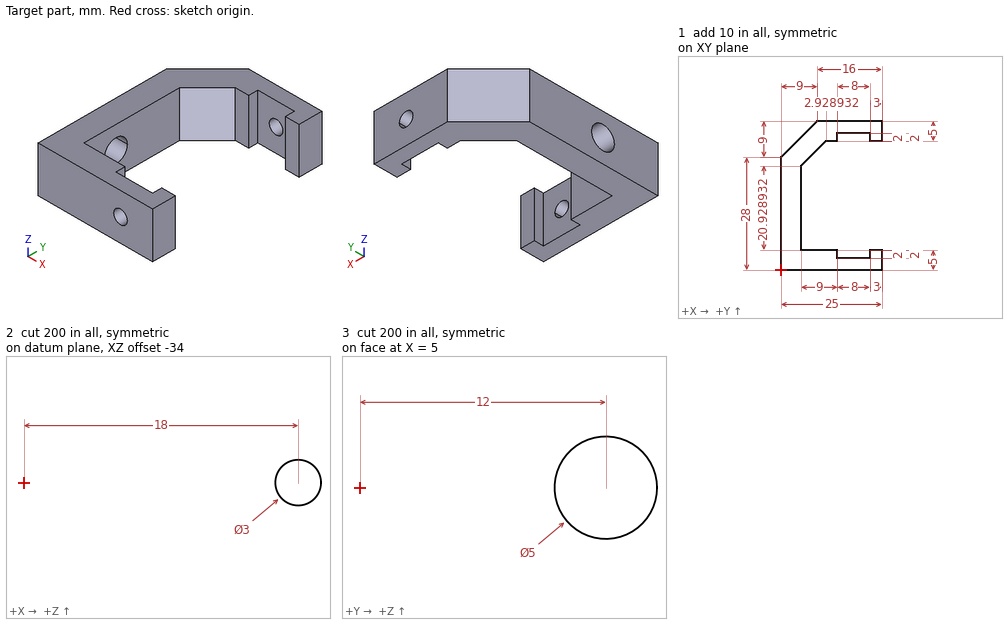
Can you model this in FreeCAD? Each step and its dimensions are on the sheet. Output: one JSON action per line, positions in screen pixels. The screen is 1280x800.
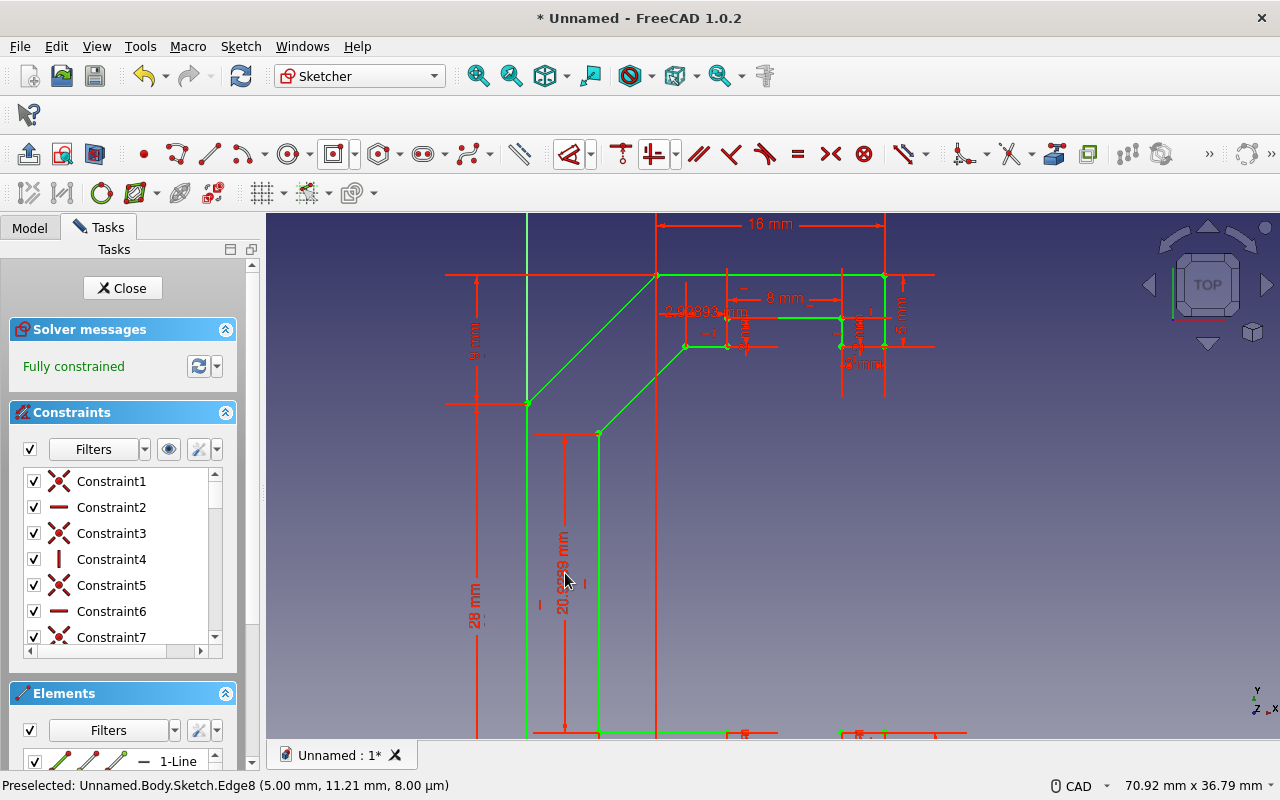
{"action": "left_click", "coordinate": [123, 288]}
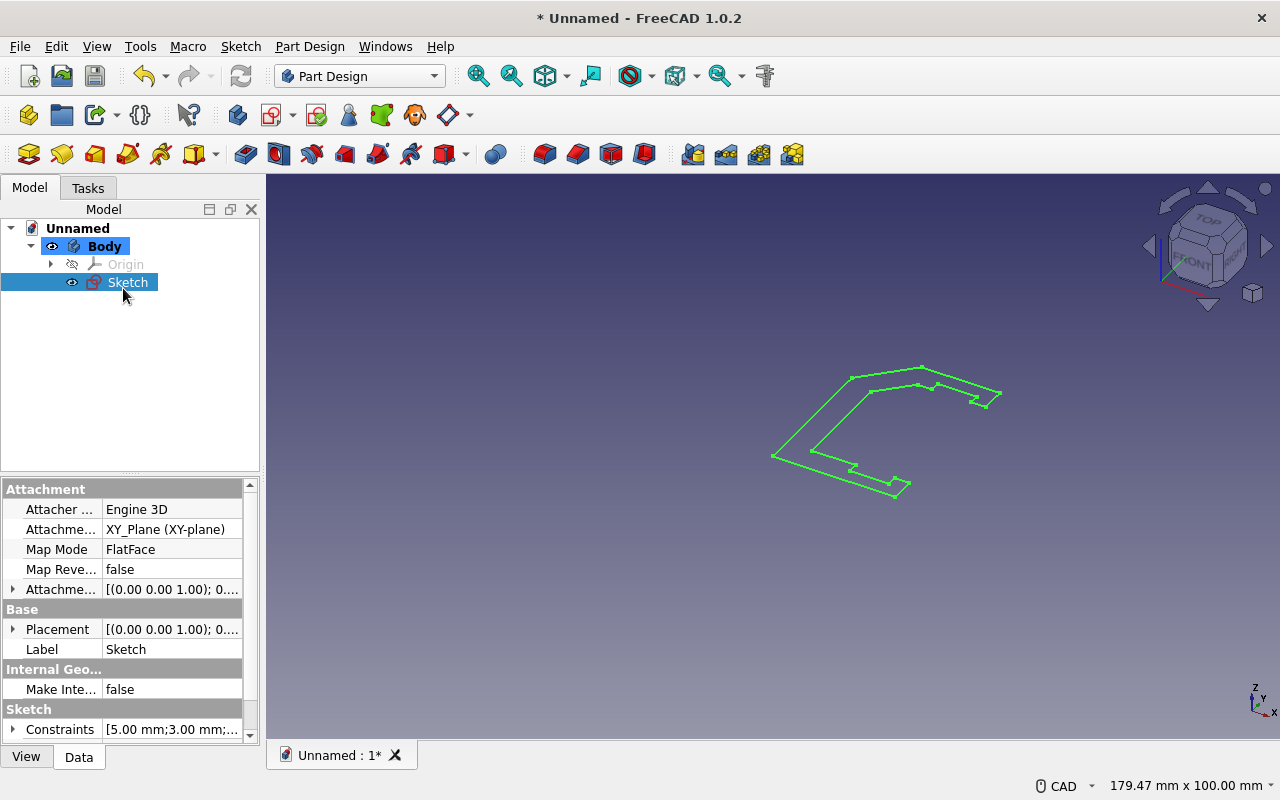
{"action": "left_click", "coordinate": [29, 154]}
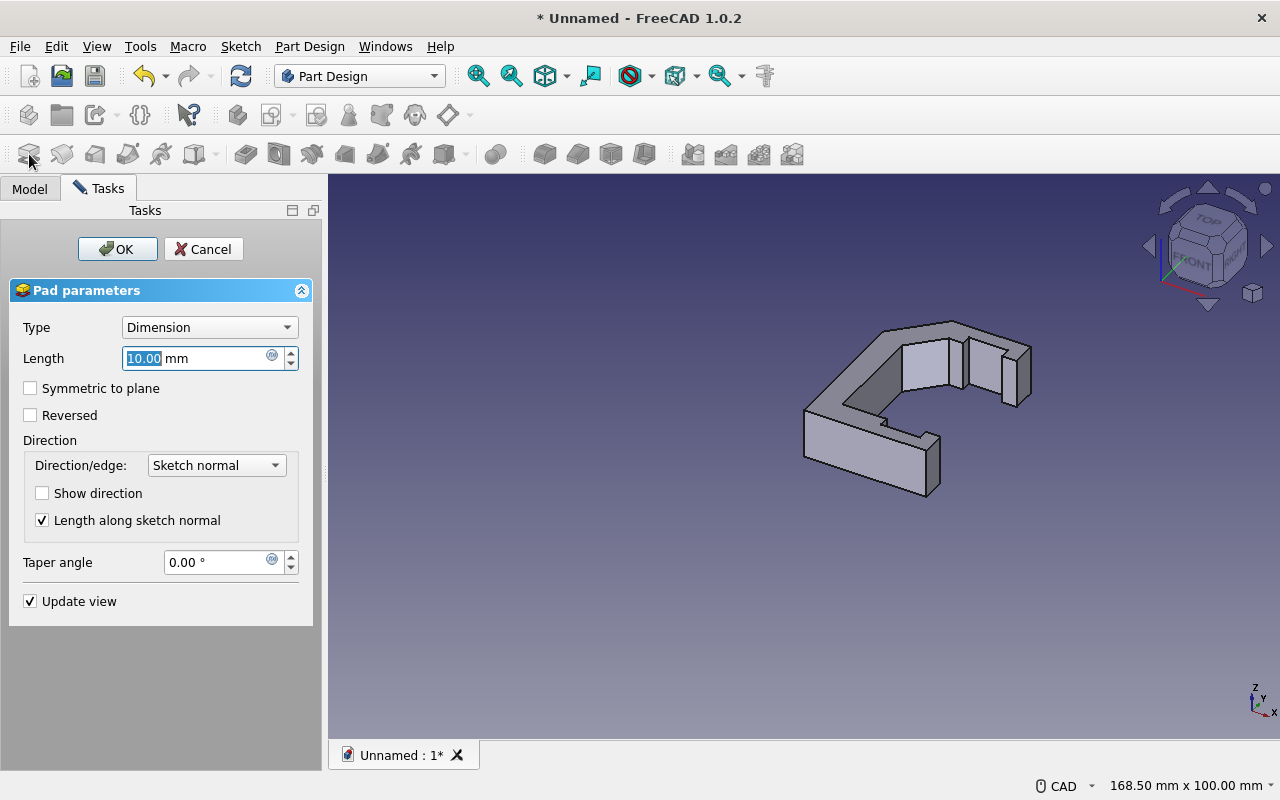
{"action": "type", "text": "10"}
{"action": "key", "text": "Tab"}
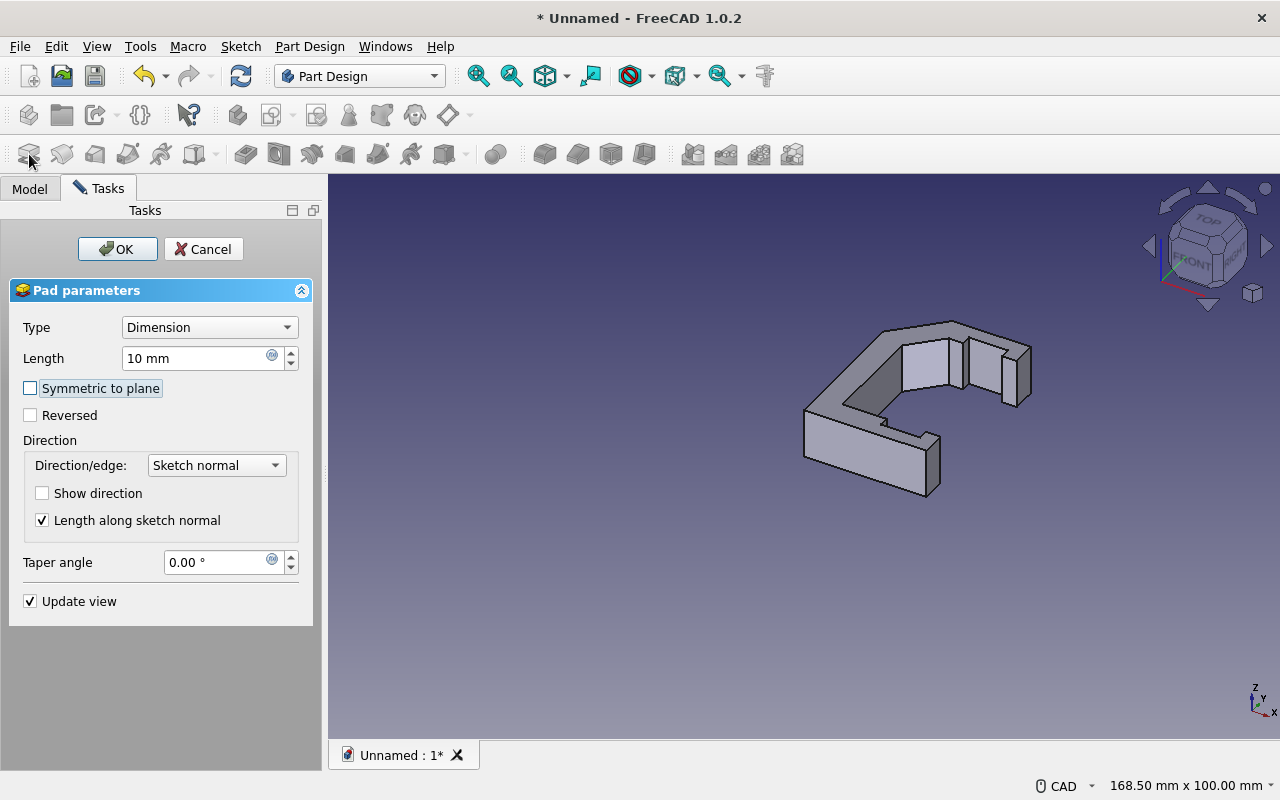
{"action": "left_click", "coordinate": [31, 388]}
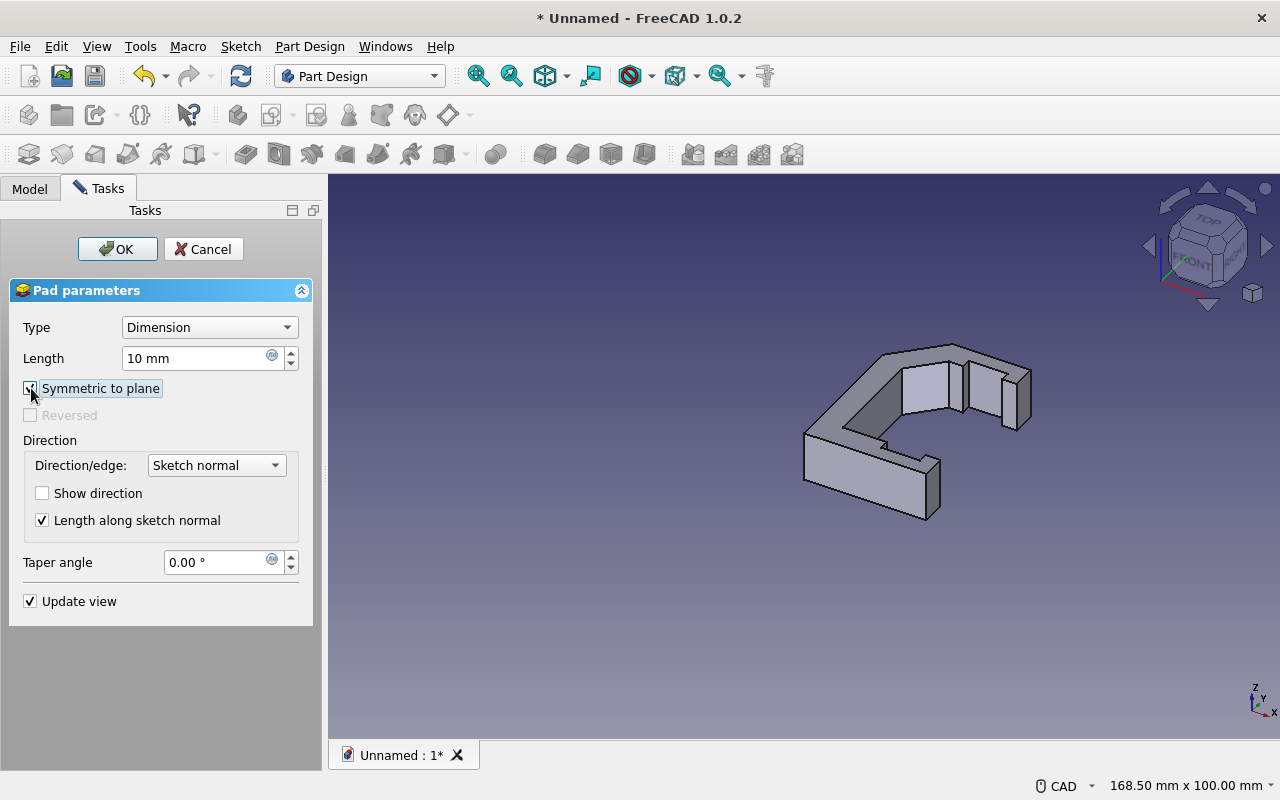
{"action": "left_click", "coordinate": [118, 249]}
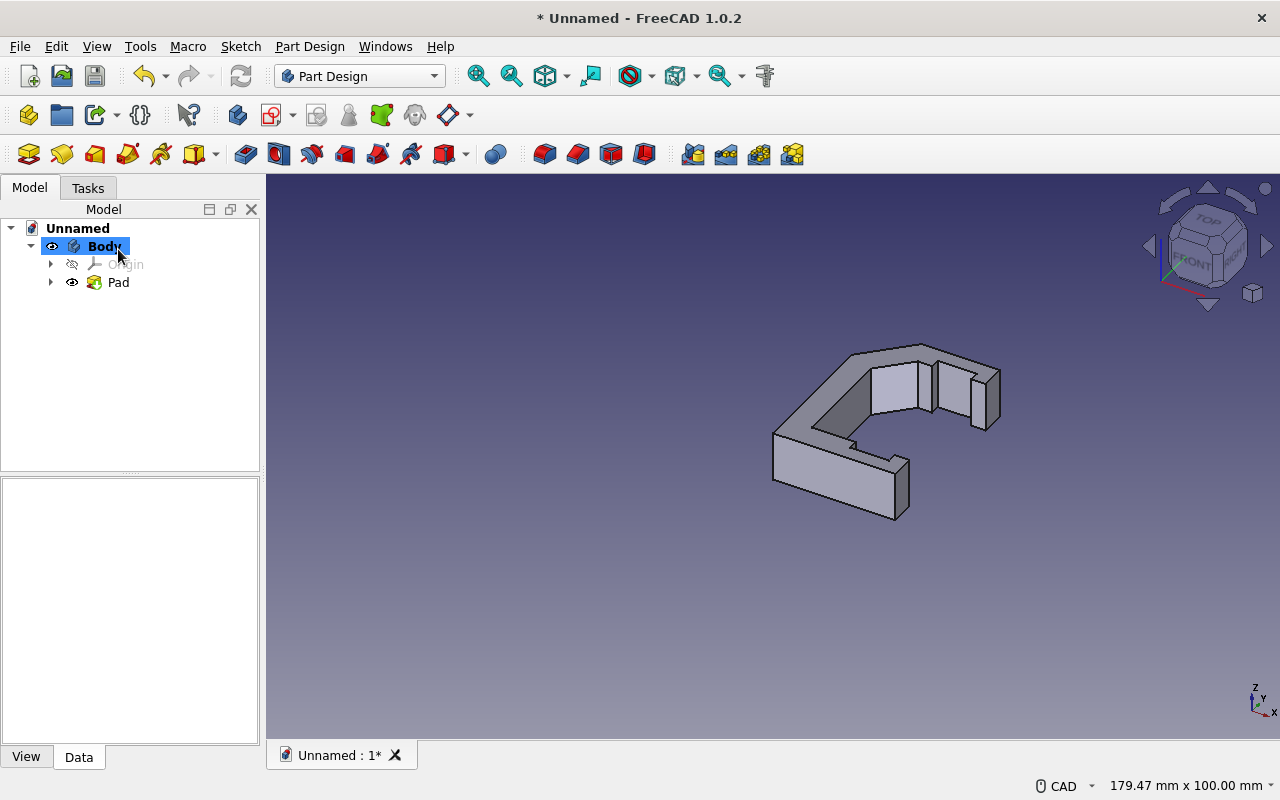
{"action": "left_click", "coordinate": [479, 76]}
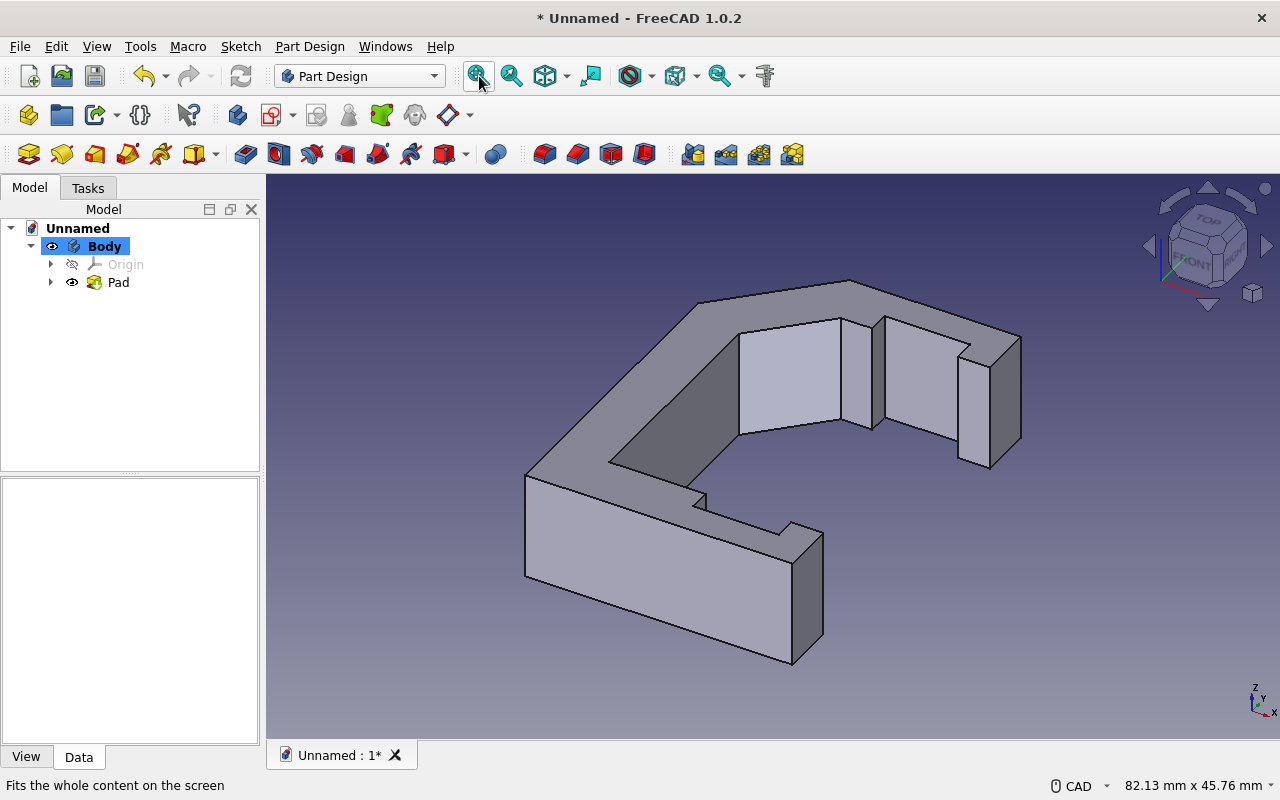
{"action": "left_click", "coordinate": [51, 264]}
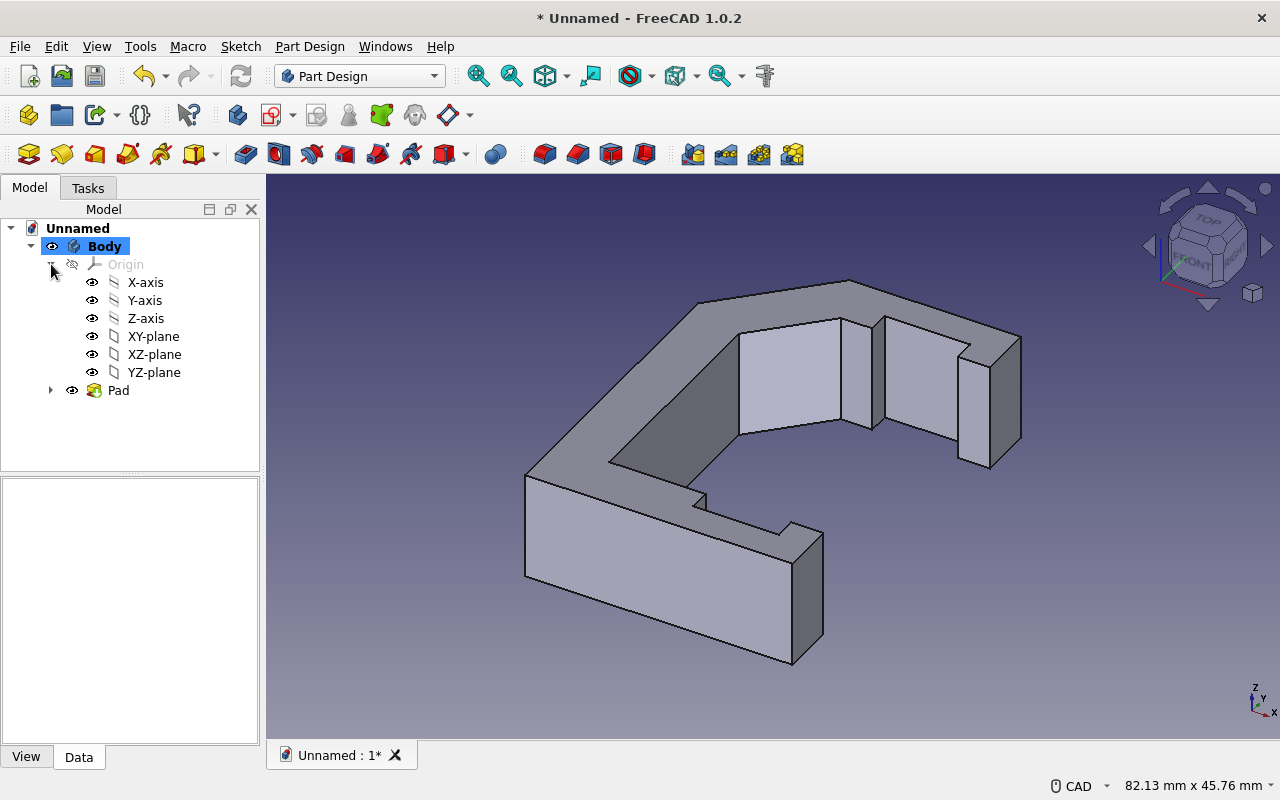
{"action": "left_click", "coordinate": [137, 354]}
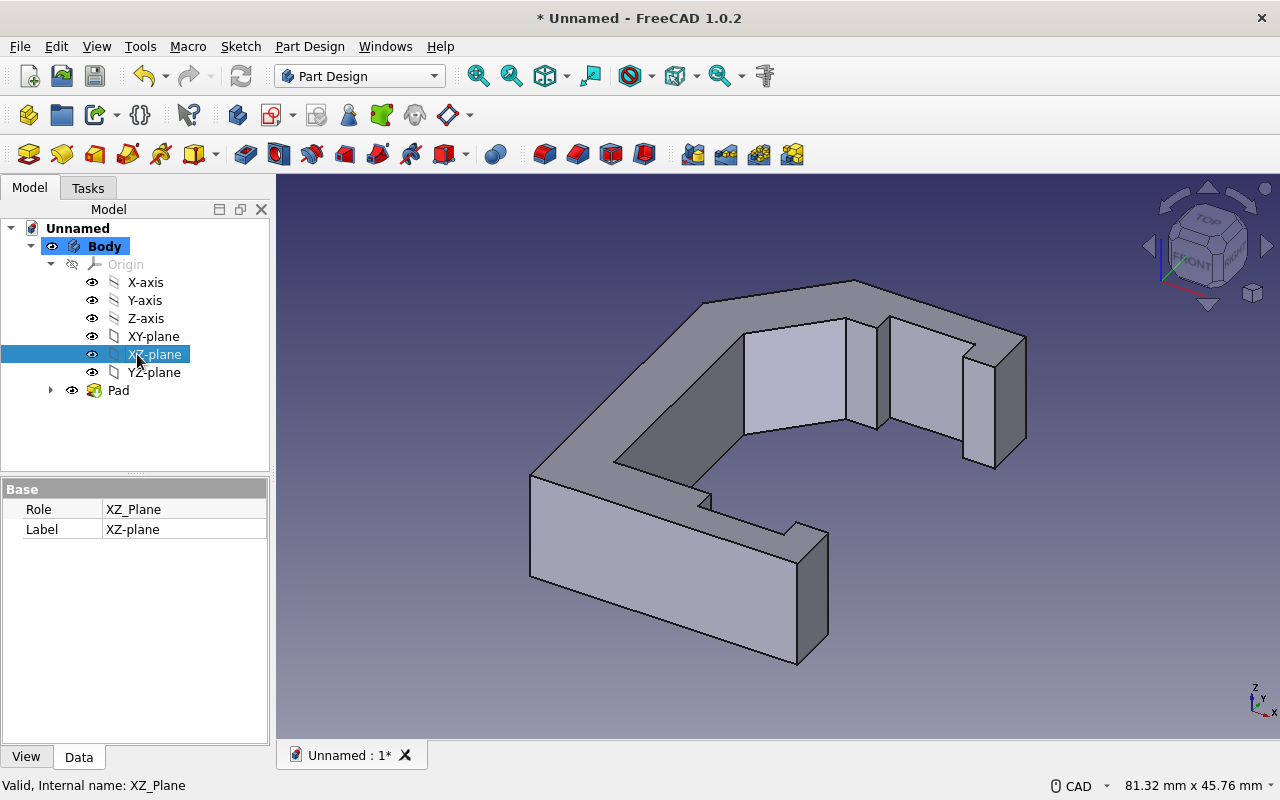
{"action": "left_click", "coordinate": [448, 116]}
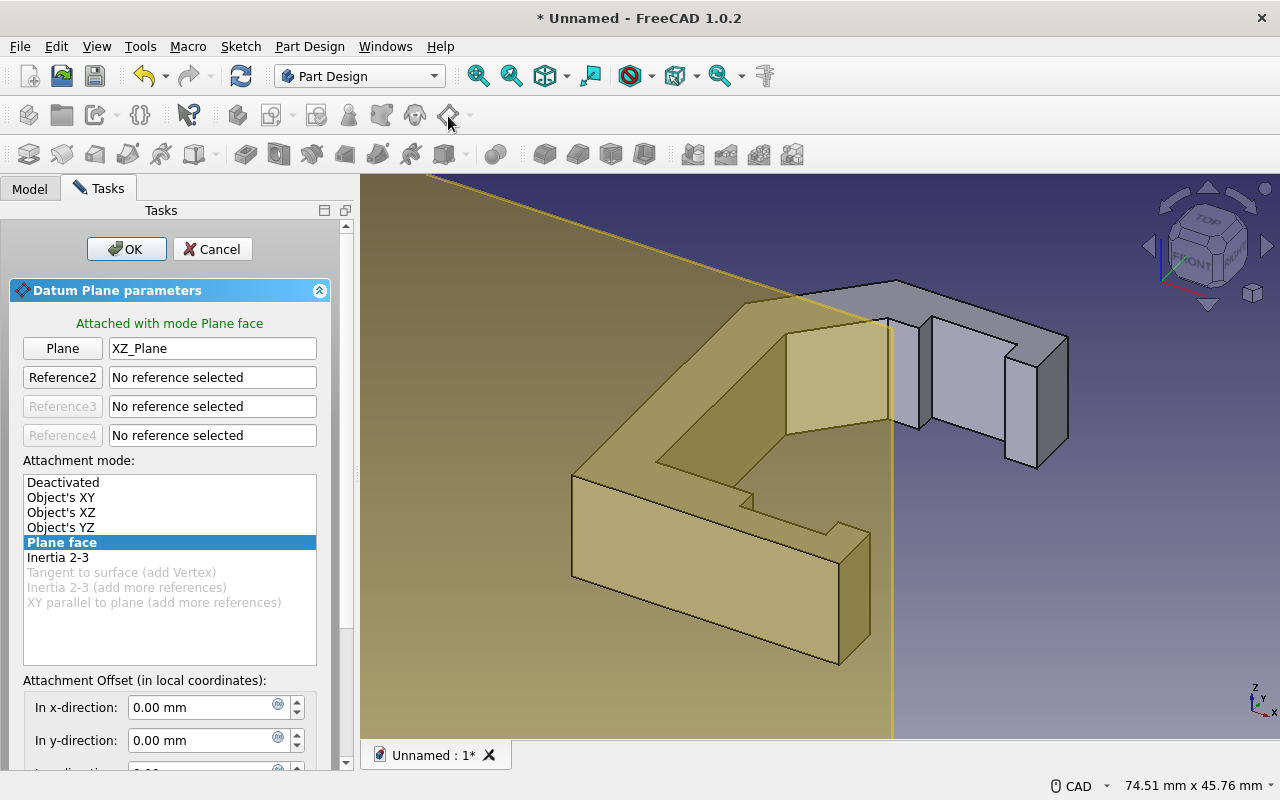
{"action": "scroll", "coordinate": [346, 495], "scroll_direction": "down", "scroll_amount": 2}